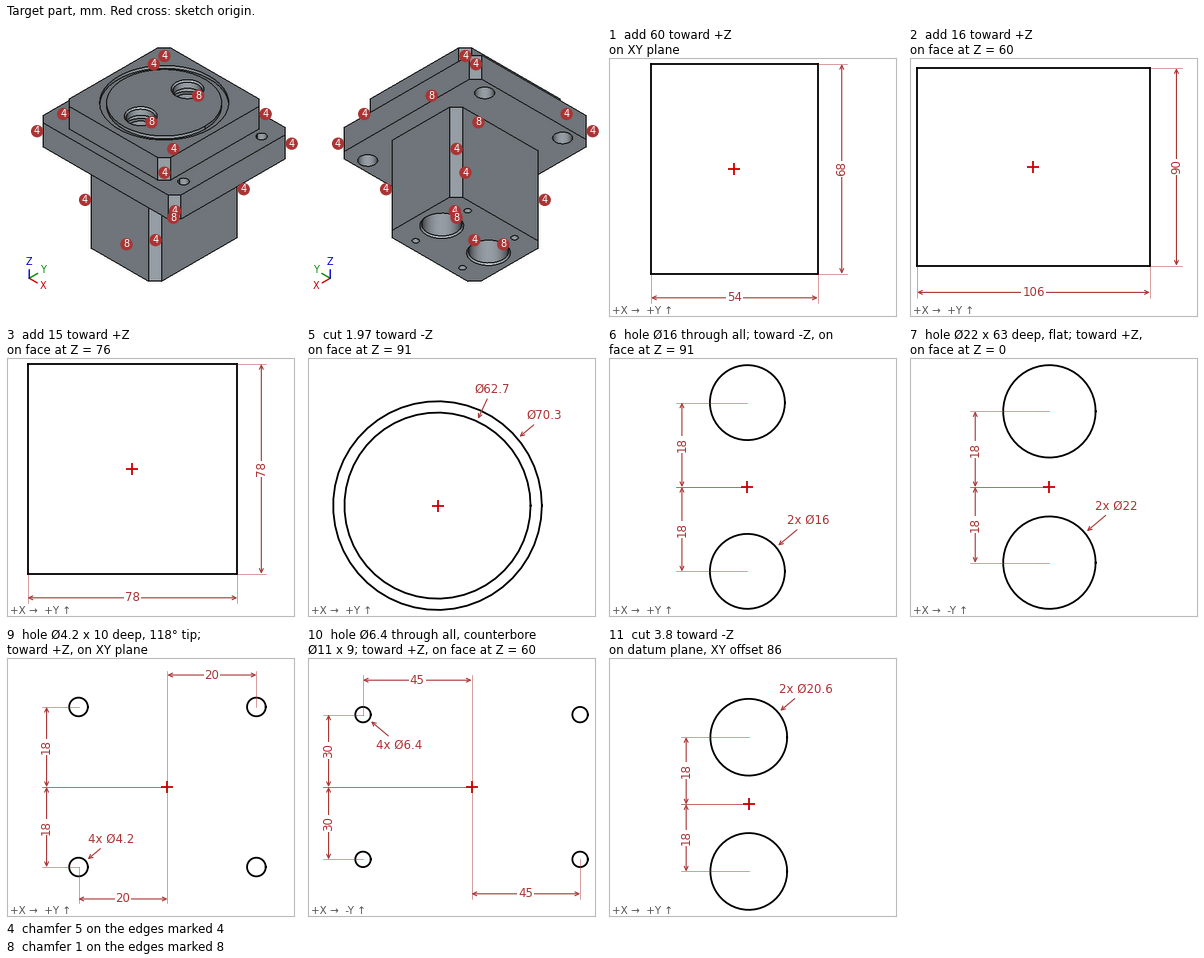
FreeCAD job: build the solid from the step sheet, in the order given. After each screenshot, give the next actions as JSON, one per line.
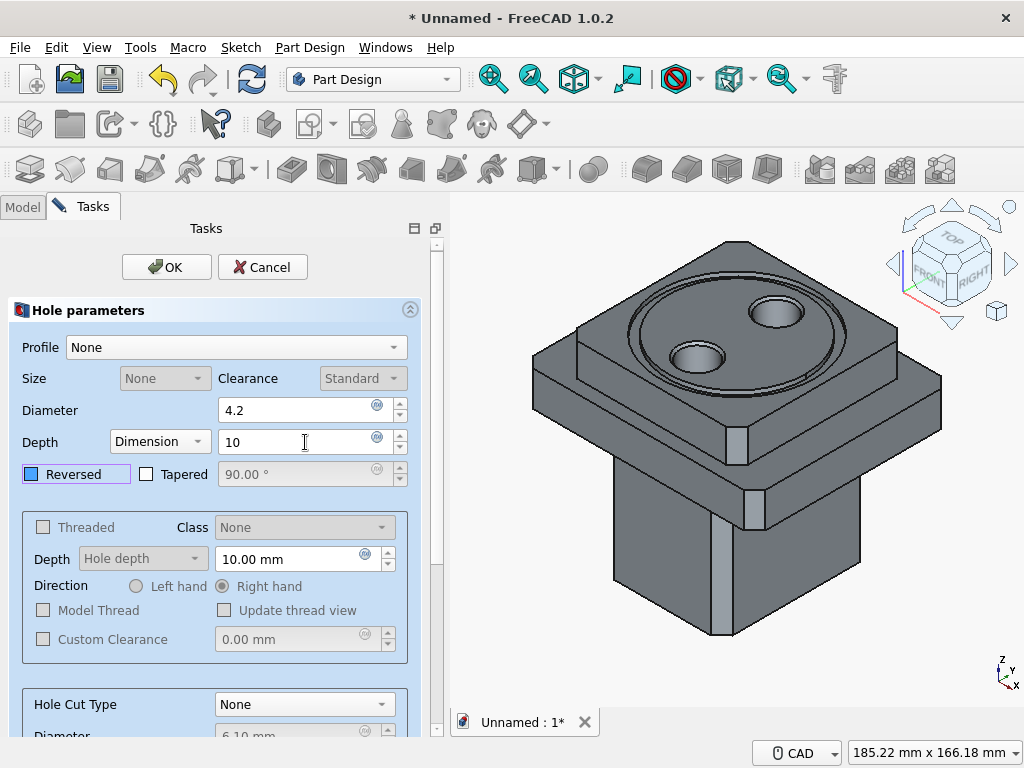
{"action": "left_click", "coordinate": [30, 474]}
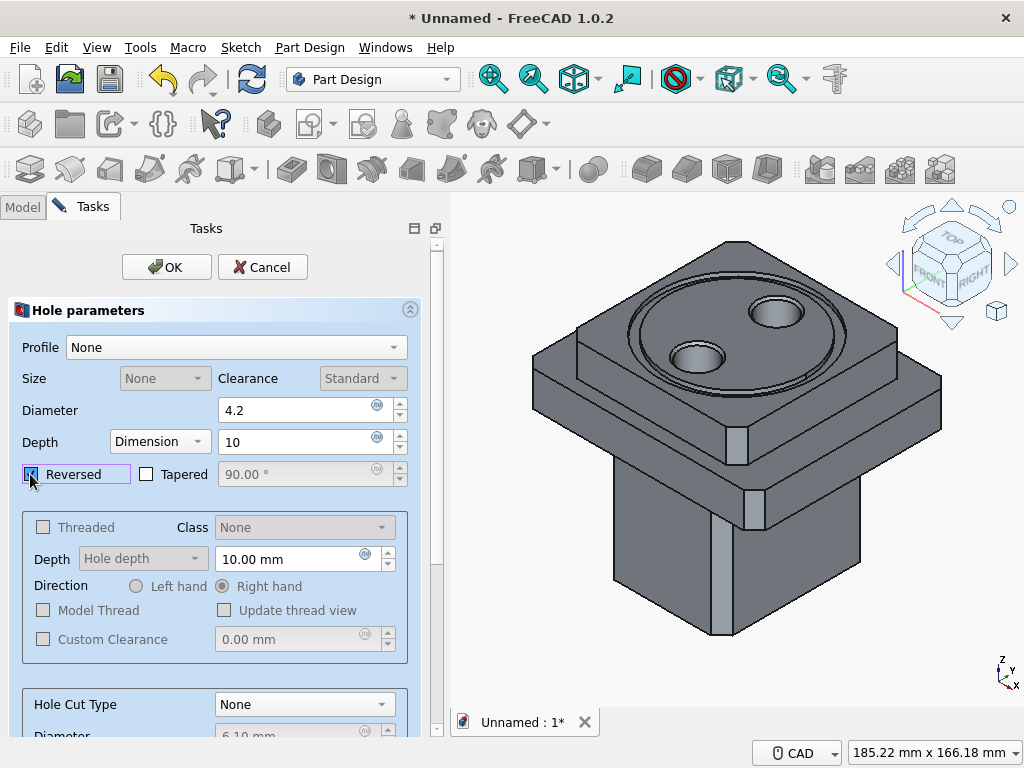
{"action": "left_click", "coordinate": [167, 267]}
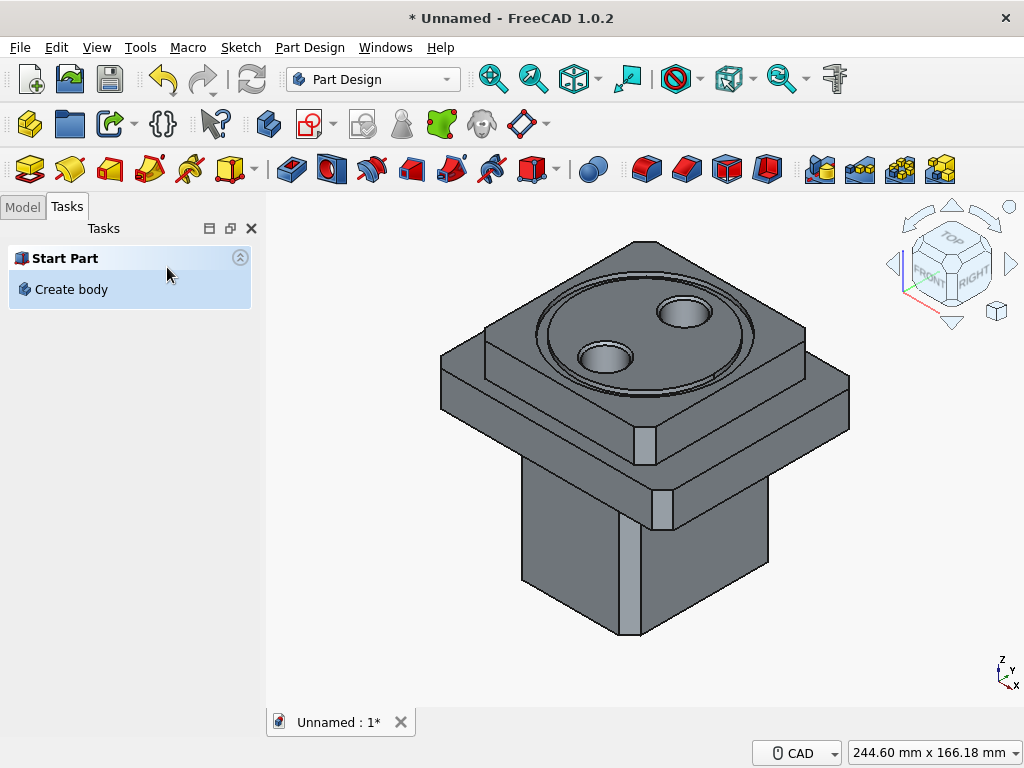
{"action": "key", "text": "5"}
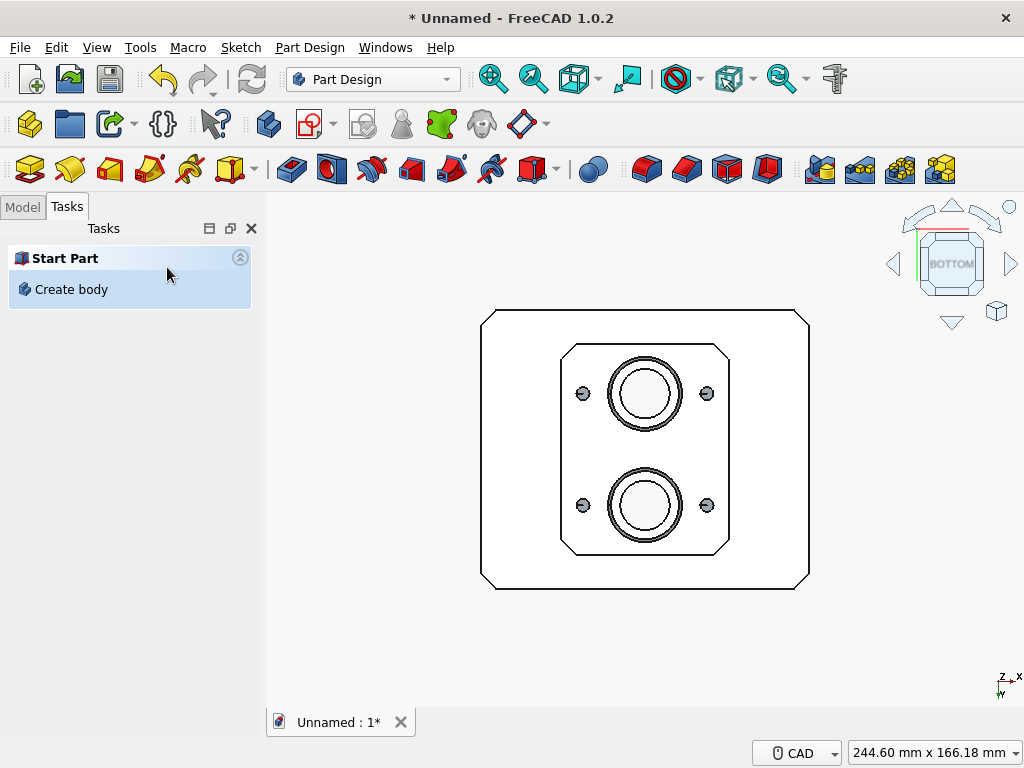
{"action": "left_click", "coordinate": [786, 528]}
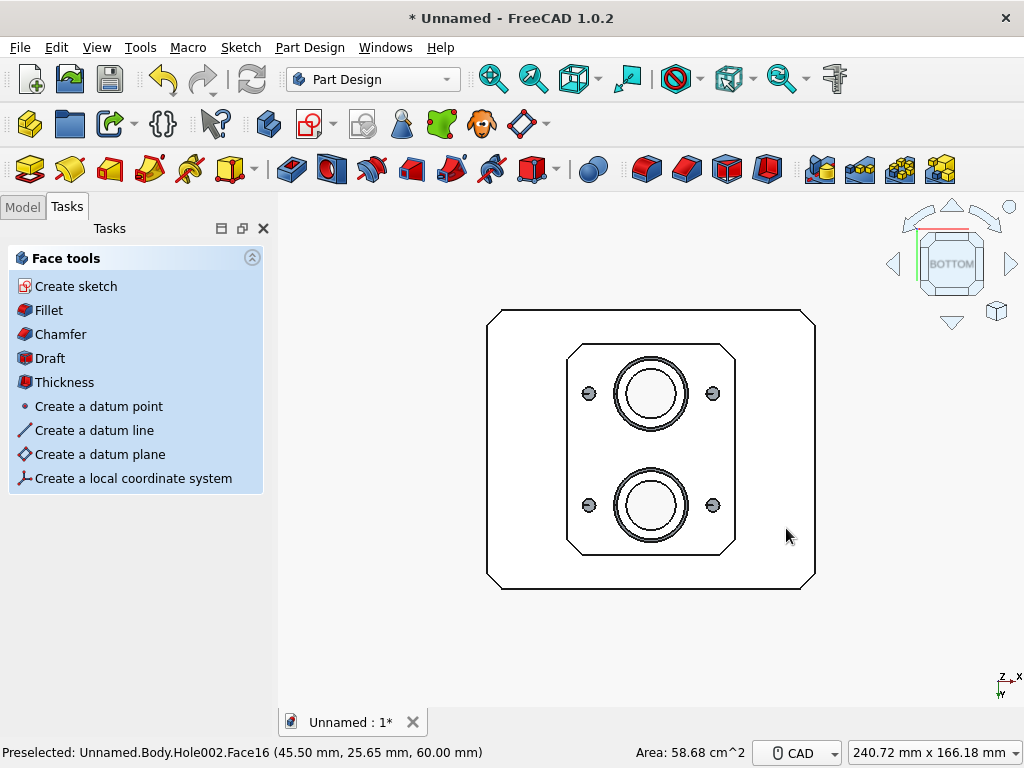
{"action": "left_click", "coordinate": [310, 124]}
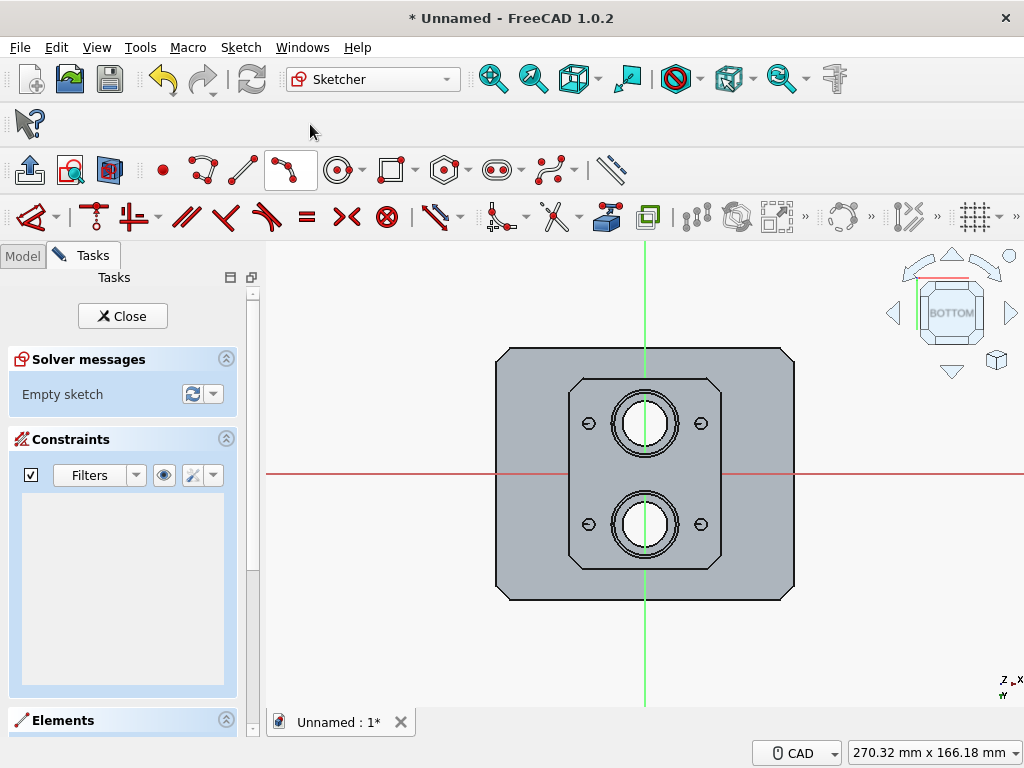
{"action": "scroll", "coordinate": [784, 474], "scroll_direction": "up", "scroll_amount": 2}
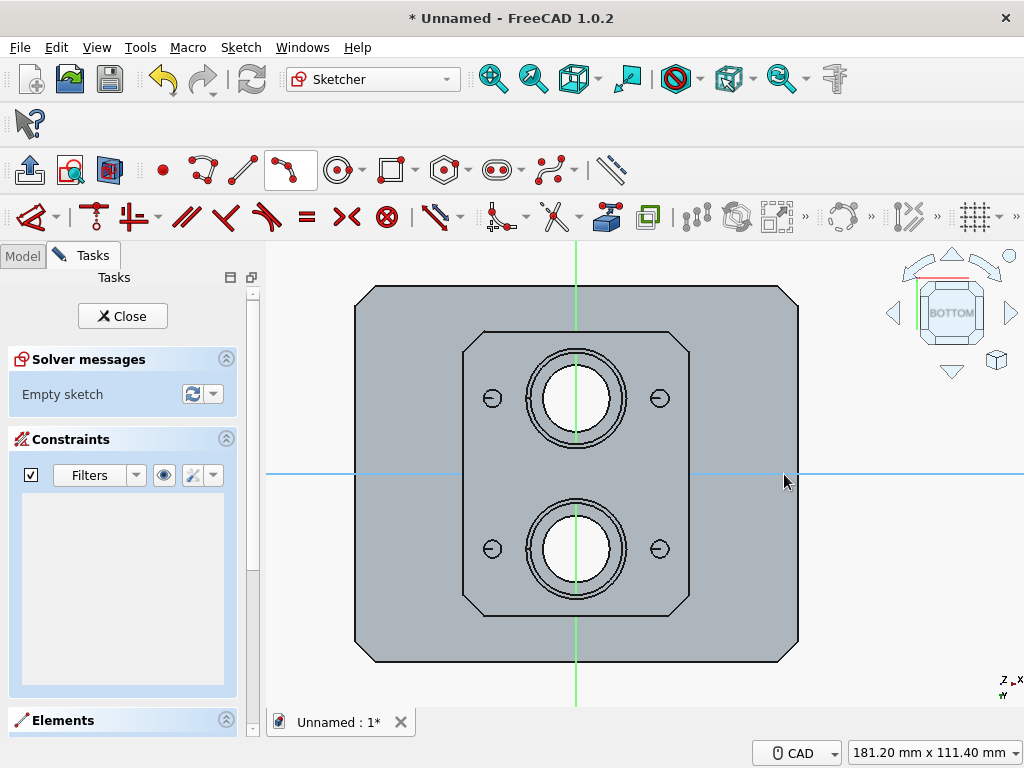
{"action": "key", "text": "g c"}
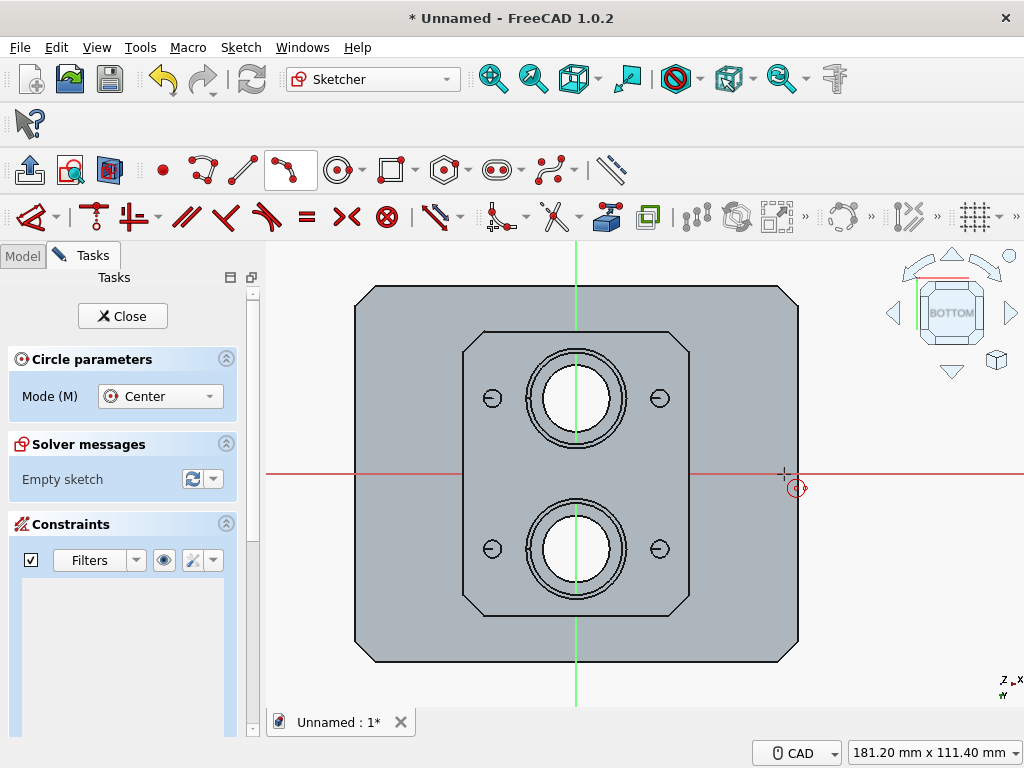
{"action": "scroll", "coordinate": [388, 348], "scroll_direction": "up", "scroll_amount": 3}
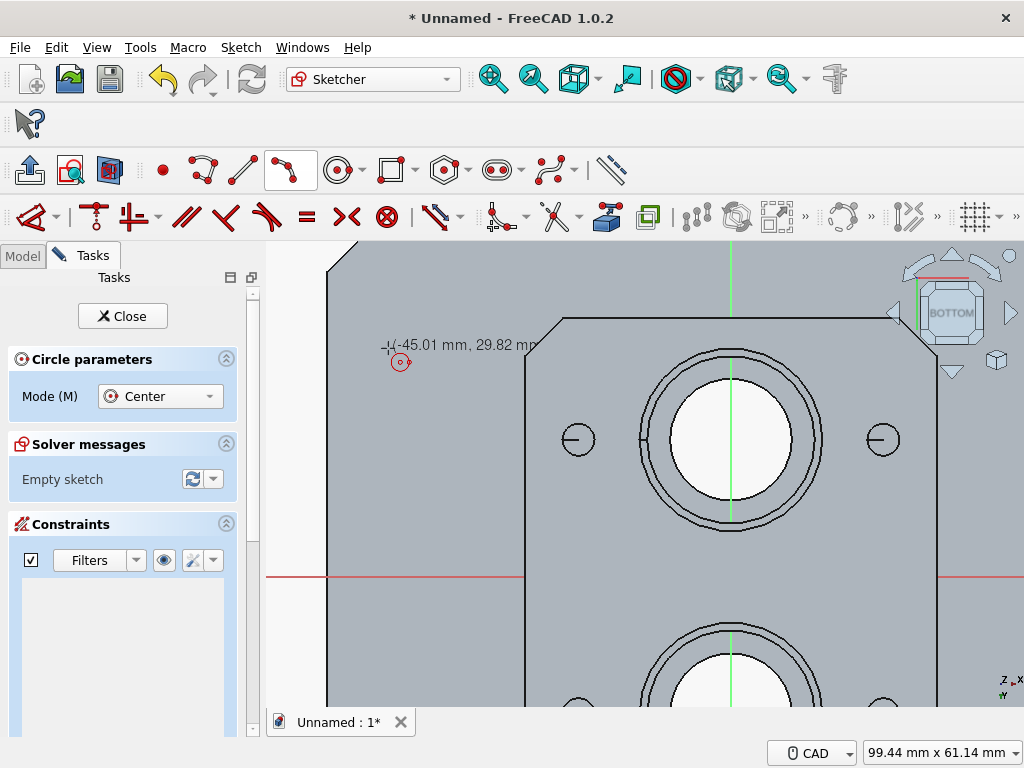
{"action": "left_click", "coordinate": [388, 348]}
{"action": "mouse_move", "coordinate": [405, 331]}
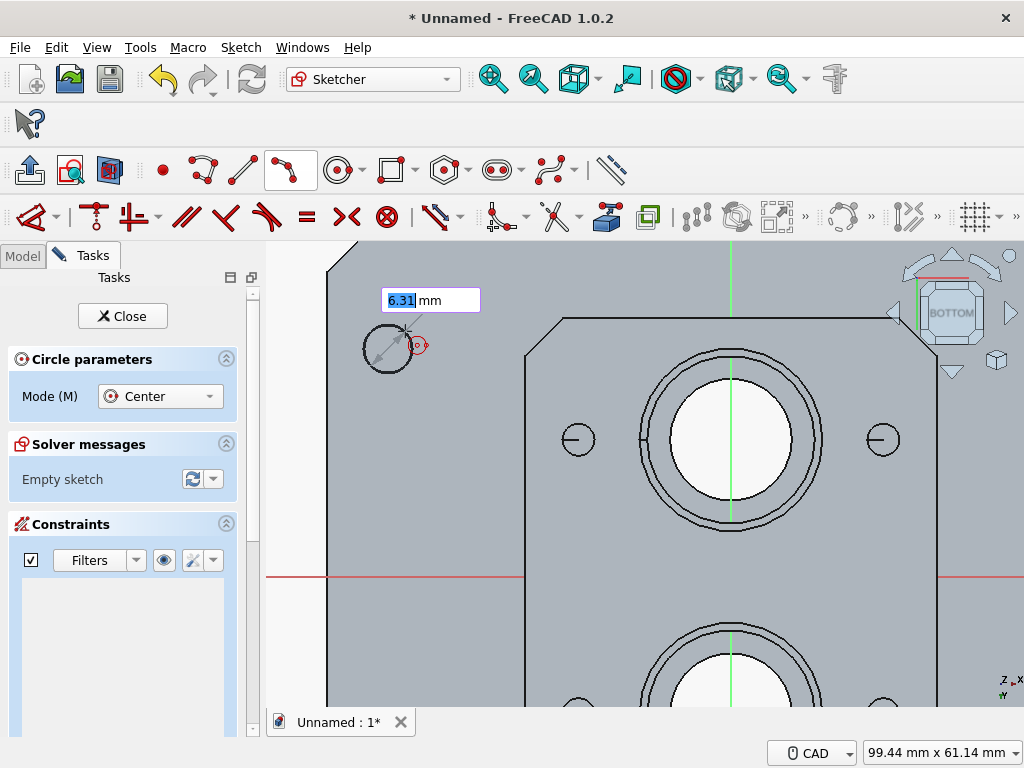
{"action": "type", "text": "6.4"}
{"action": "key", "text": "Return"}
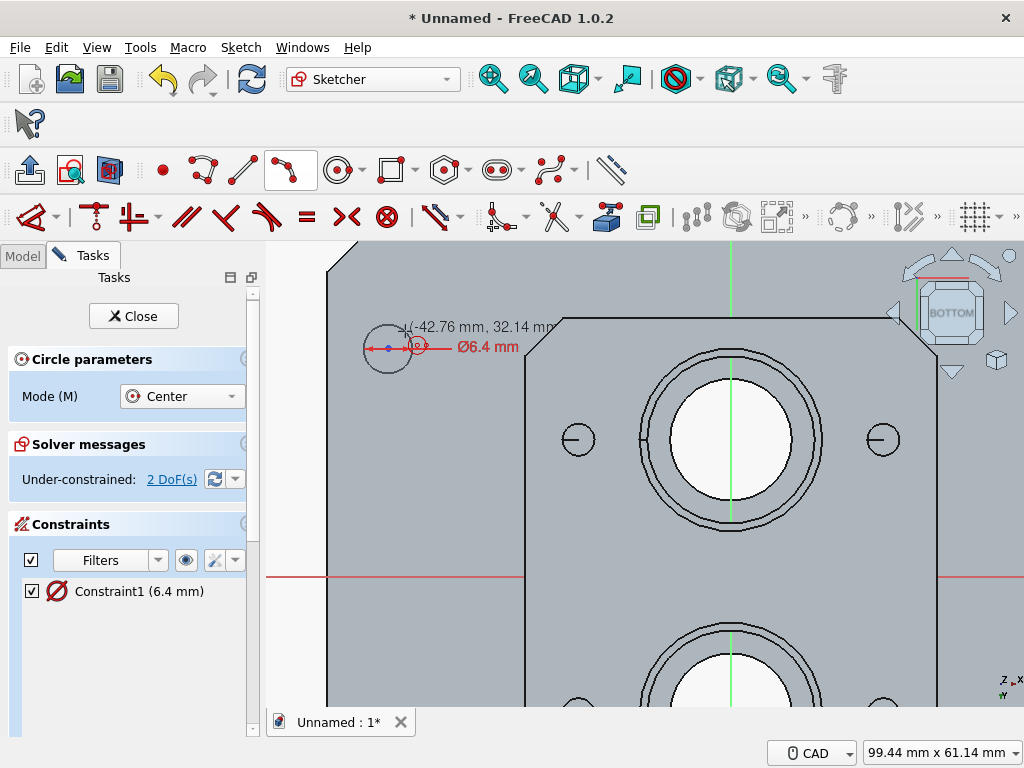
{"action": "scroll", "coordinate": [389, 349], "scroll_direction": "down", "scroll_amount": 3}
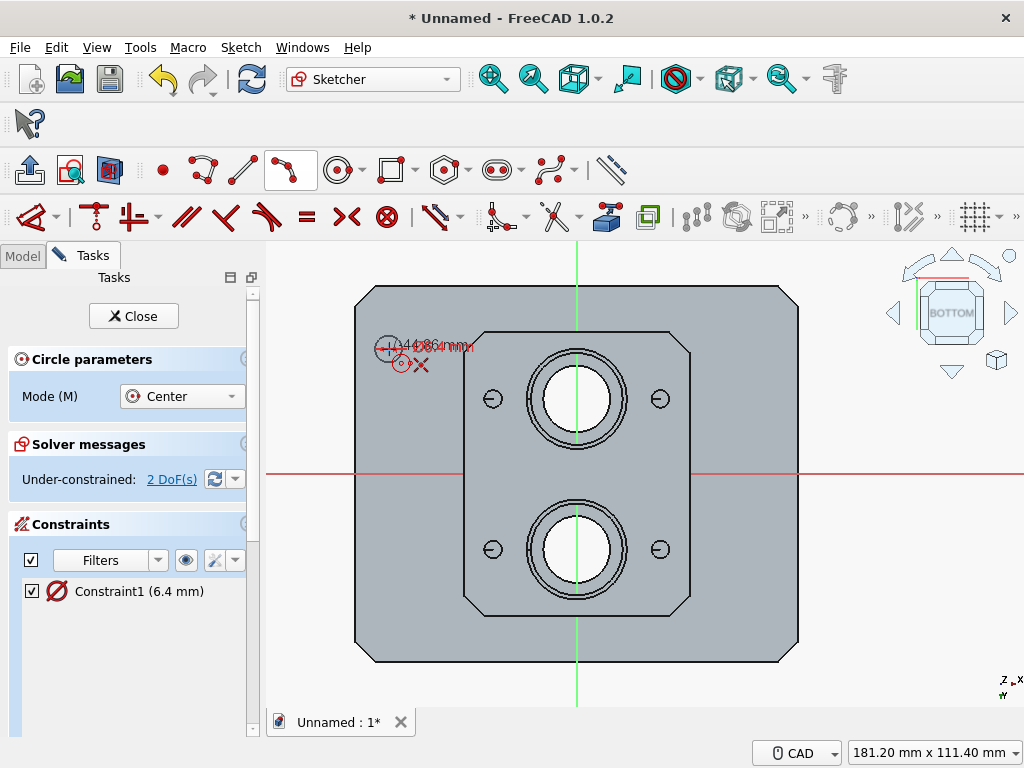
{"action": "scroll", "coordinate": [389, 600], "scroll_direction": "up", "scroll_amount": 3}